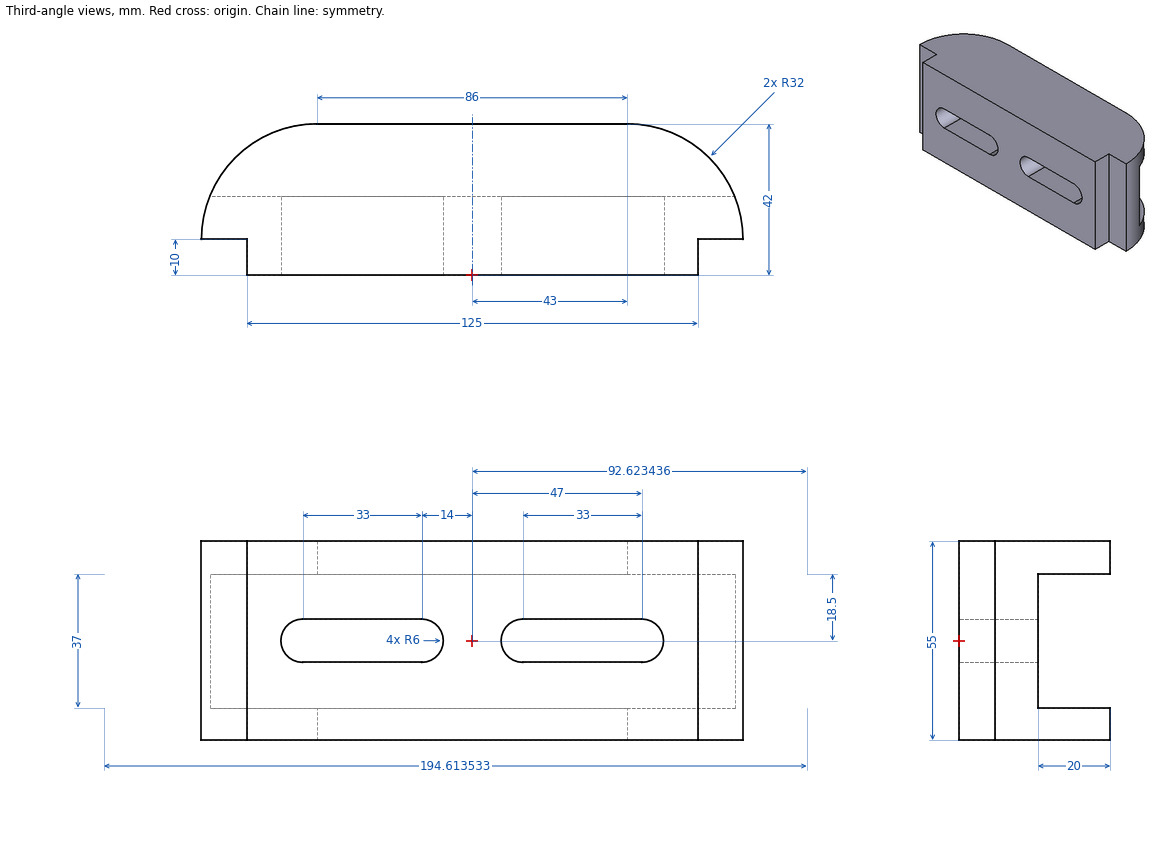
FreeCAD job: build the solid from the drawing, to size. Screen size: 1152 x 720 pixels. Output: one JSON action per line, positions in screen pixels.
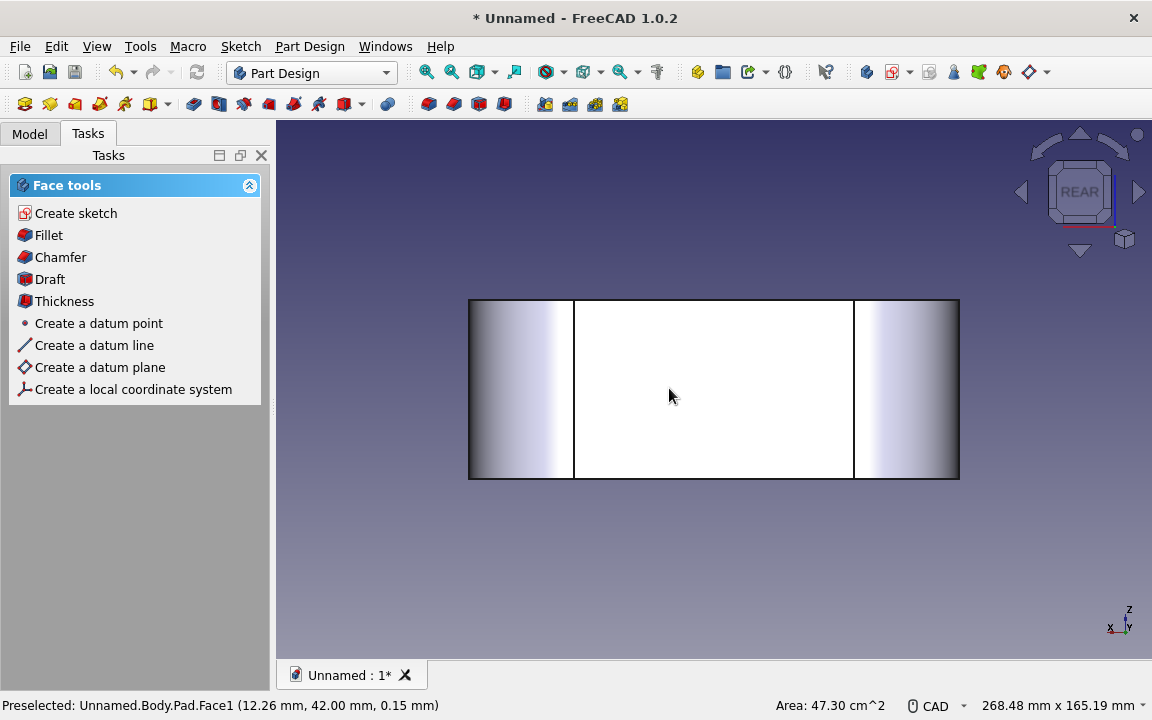
{"action": "left_click", "coordinate": [892, 72]}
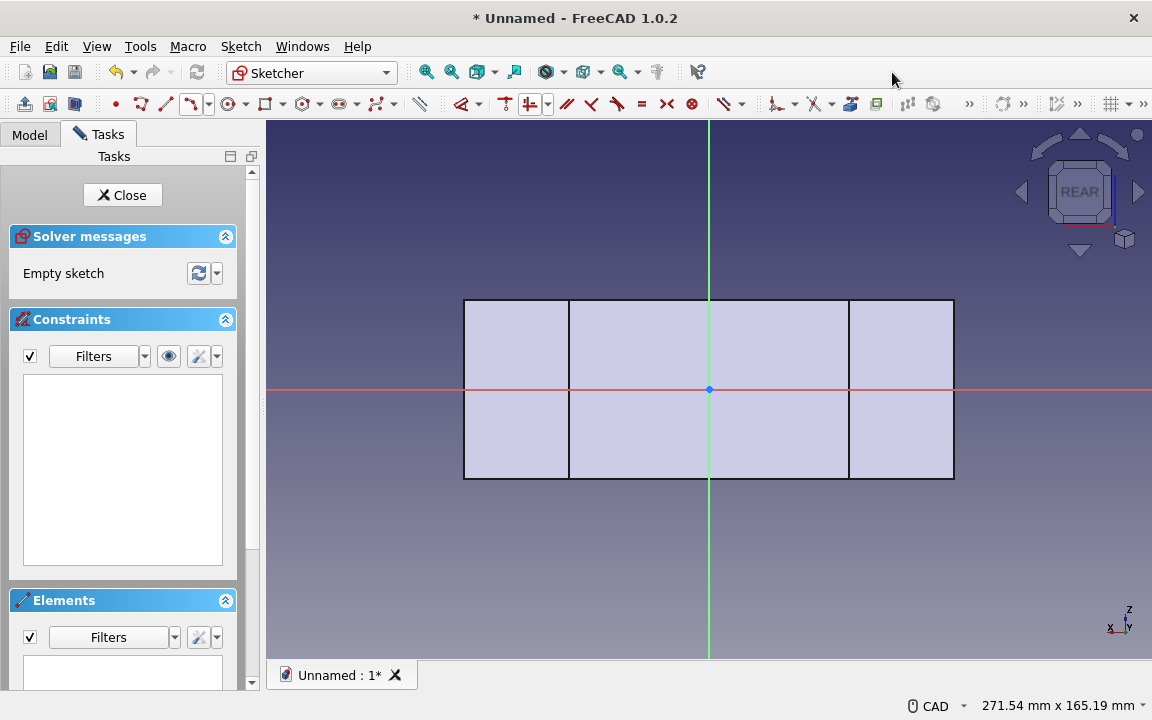
{"action": "scroll", "coordinate": [294, 390], "scroll_direction": "down", "scroll_amount": 1}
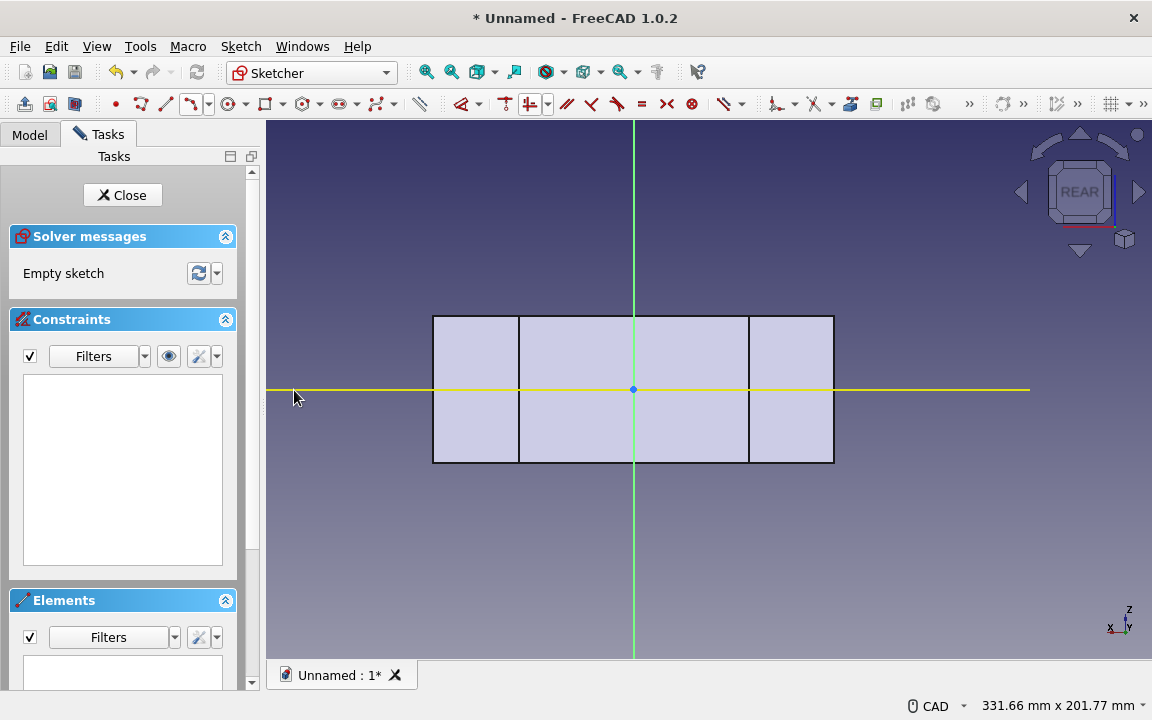
{"action": "left_click", "coordinate": [264, 104]}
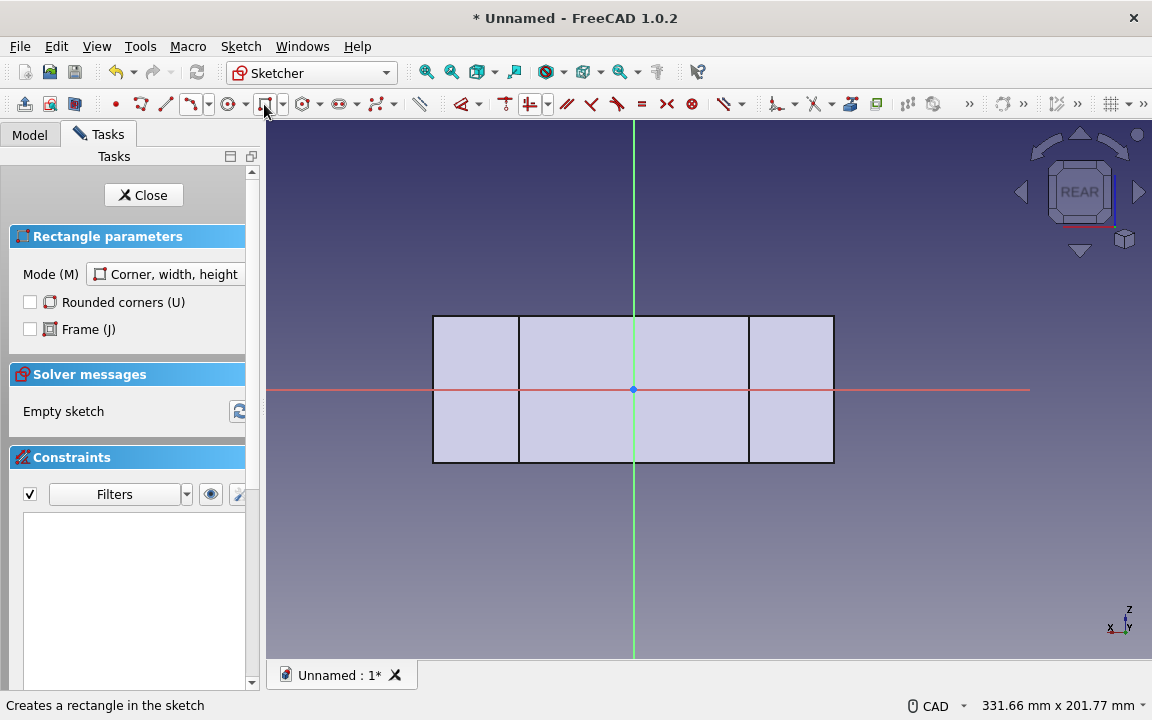
{"action": "left_click", "coordinate": [386, 340]}
{"action": "mouse_move", "coordinate": [906, 439]}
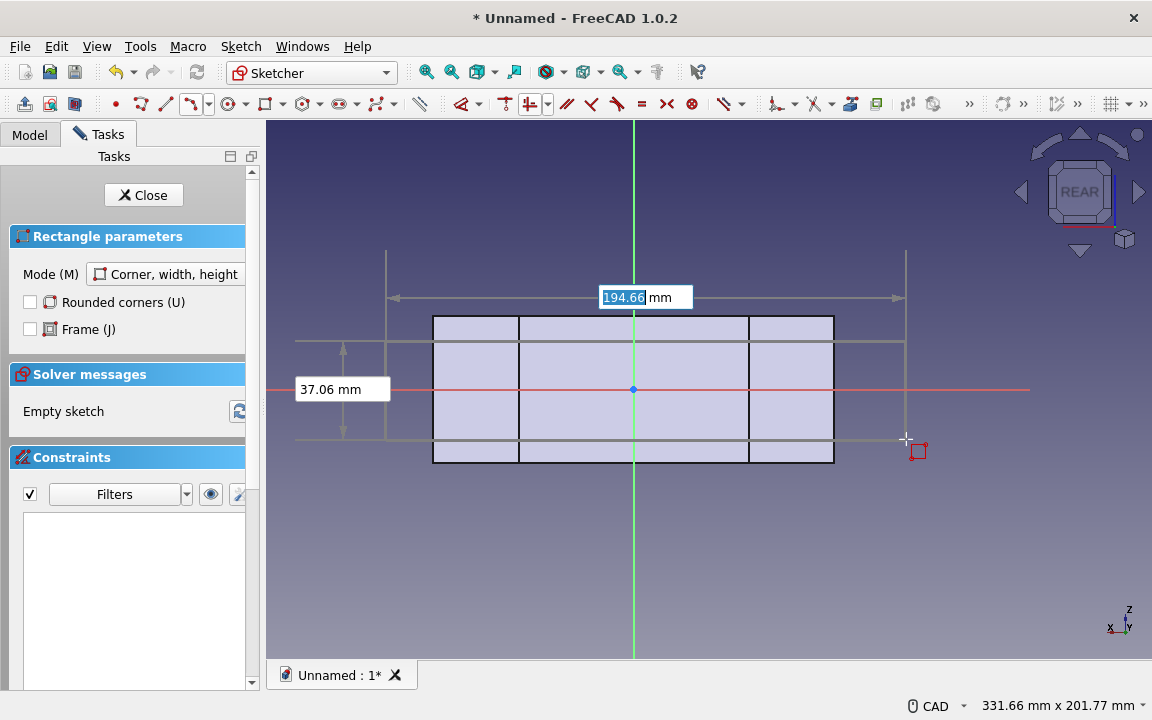
{"action": "type", "text": "194.613533"}
{"action": "key", "text": "Tab"}
{"action": "type", "text": "37"}
{"action": "key", "text": "Return"}
{"action": "key", "text": "Escape"}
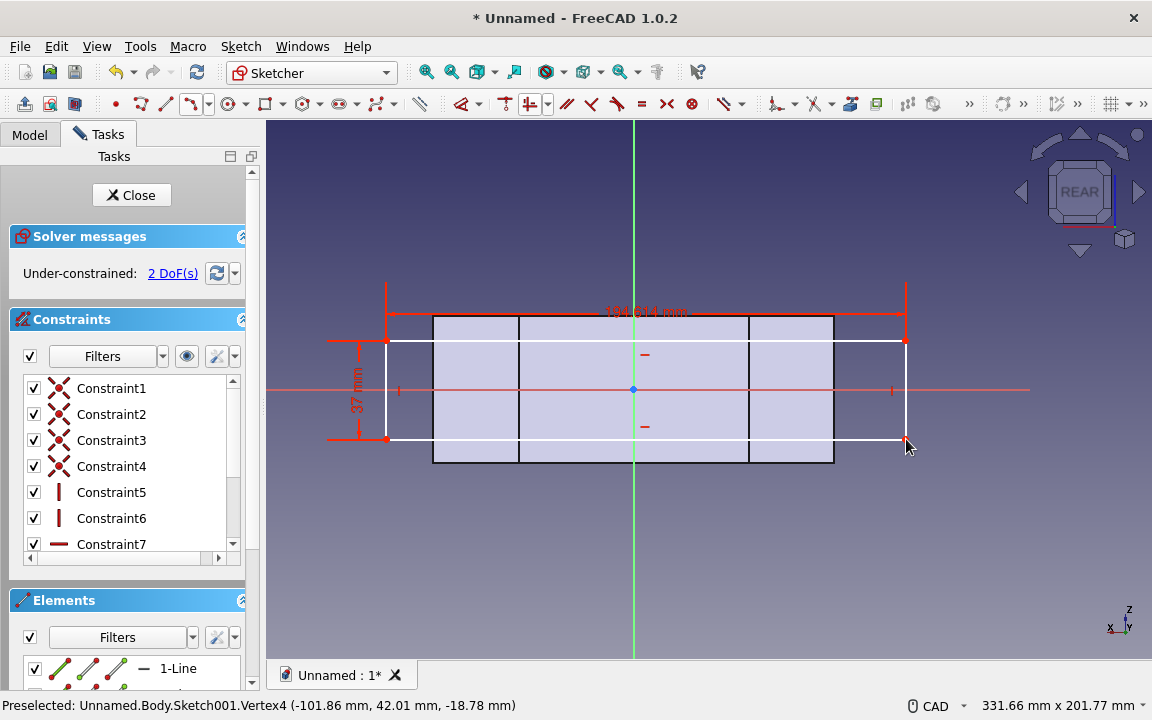
{"action": "left_click", "coordinate": [460, 104]}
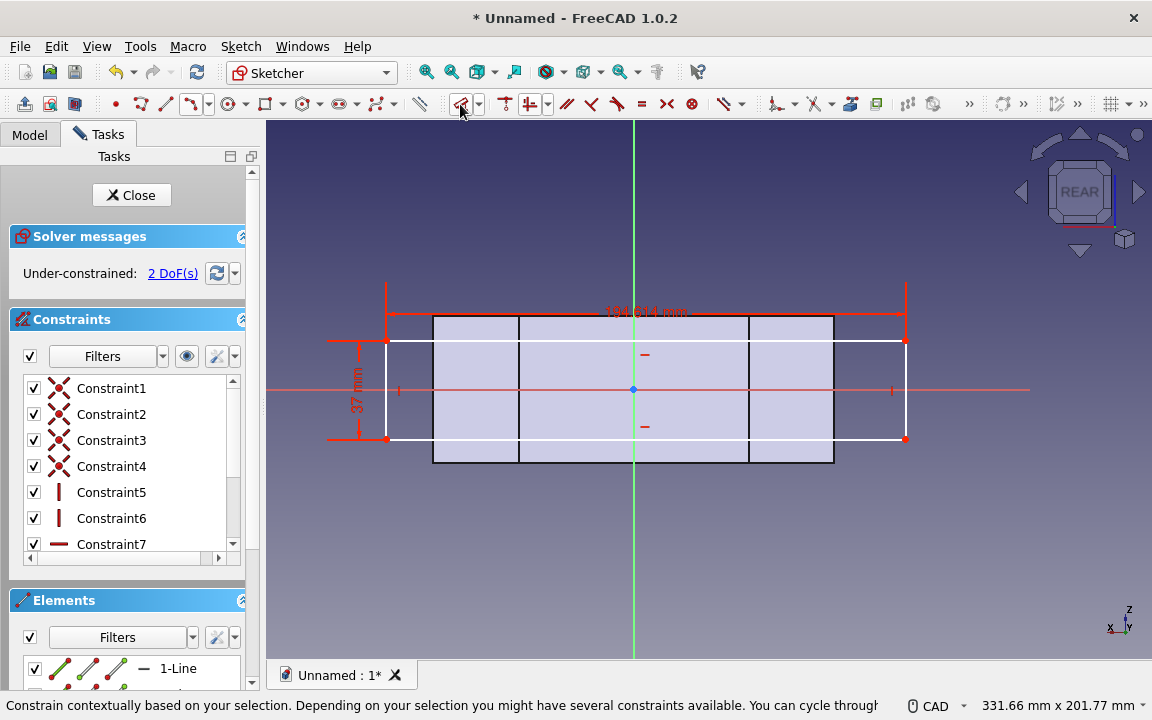
{"action": "left_click", "coordinate": [386, 341]}
{"action": "left_click", "coordinate": [352, 365]}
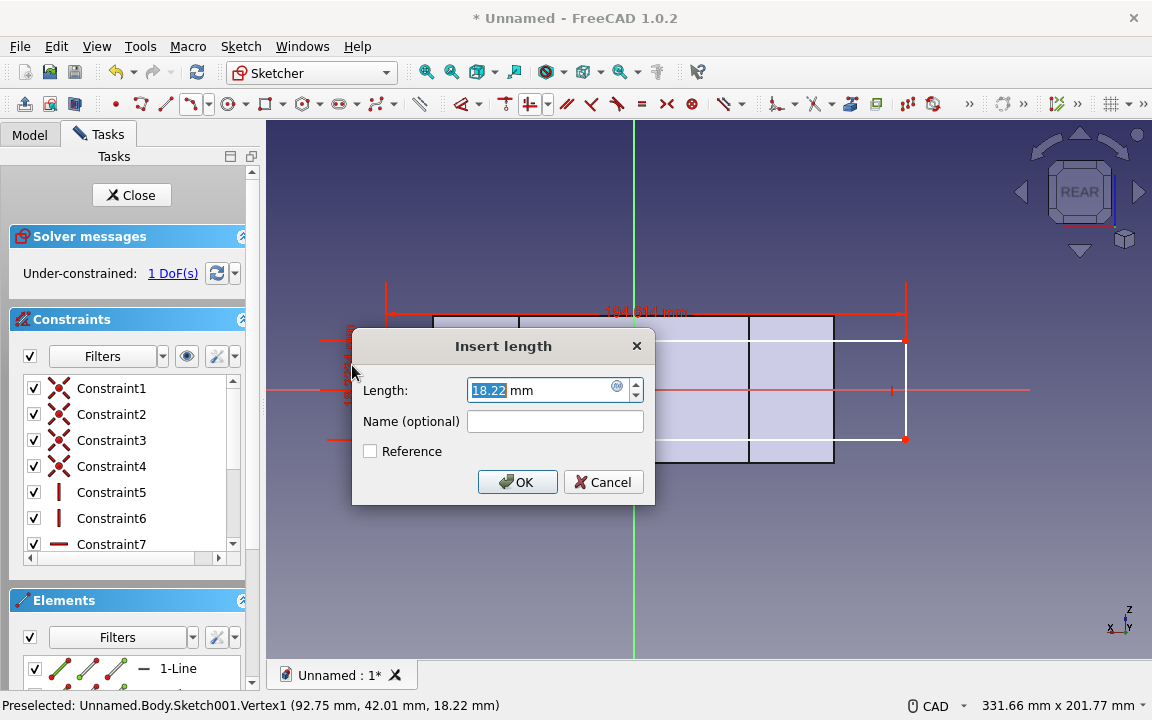
{"action": "type", "text": "18.5"}
{"action": "key", "text": "Return"}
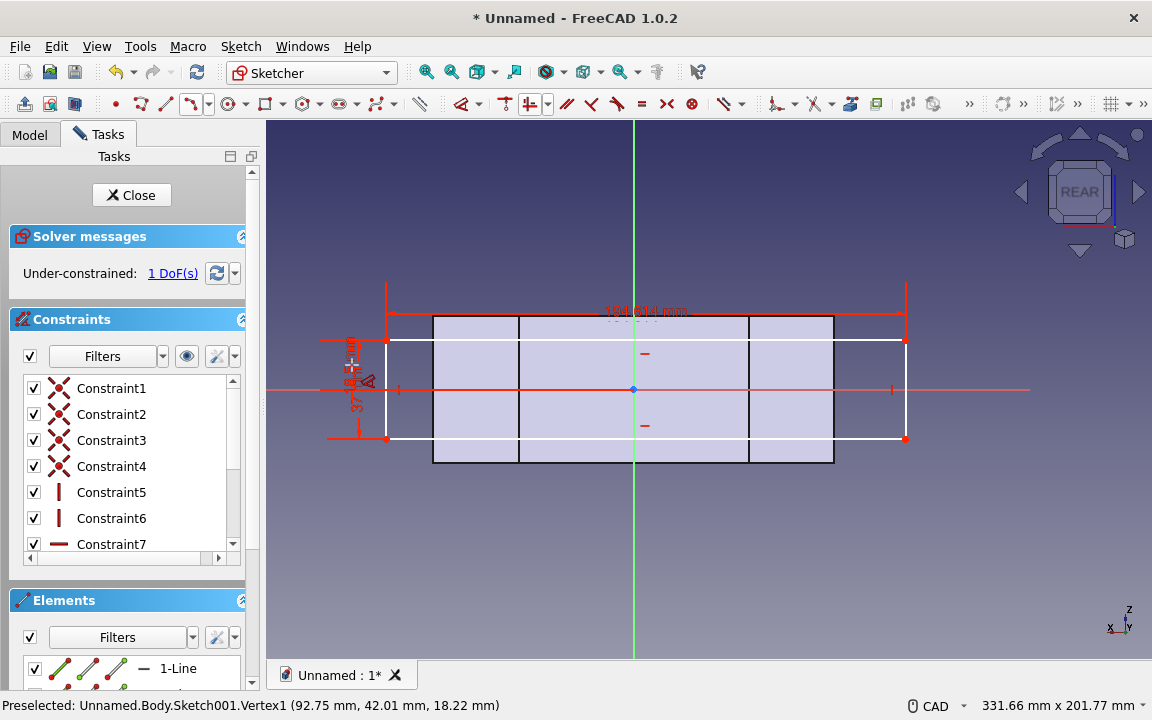
{"action": "left_click", "coordinate": [386, 340]}
{"action": "left_click", "coordinate": [510, 306]}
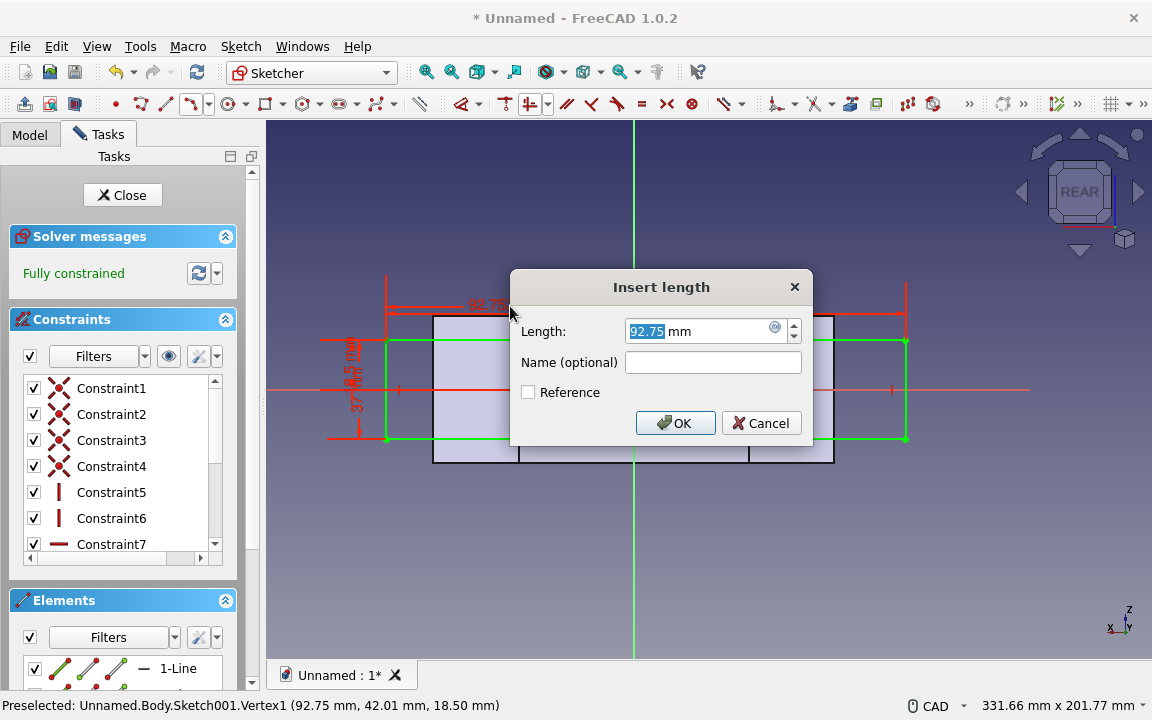
{"action": "type", "text": "92.623436"}
{"action": "key", "text": "Return"}
{"action": "key", "text": "Escape"}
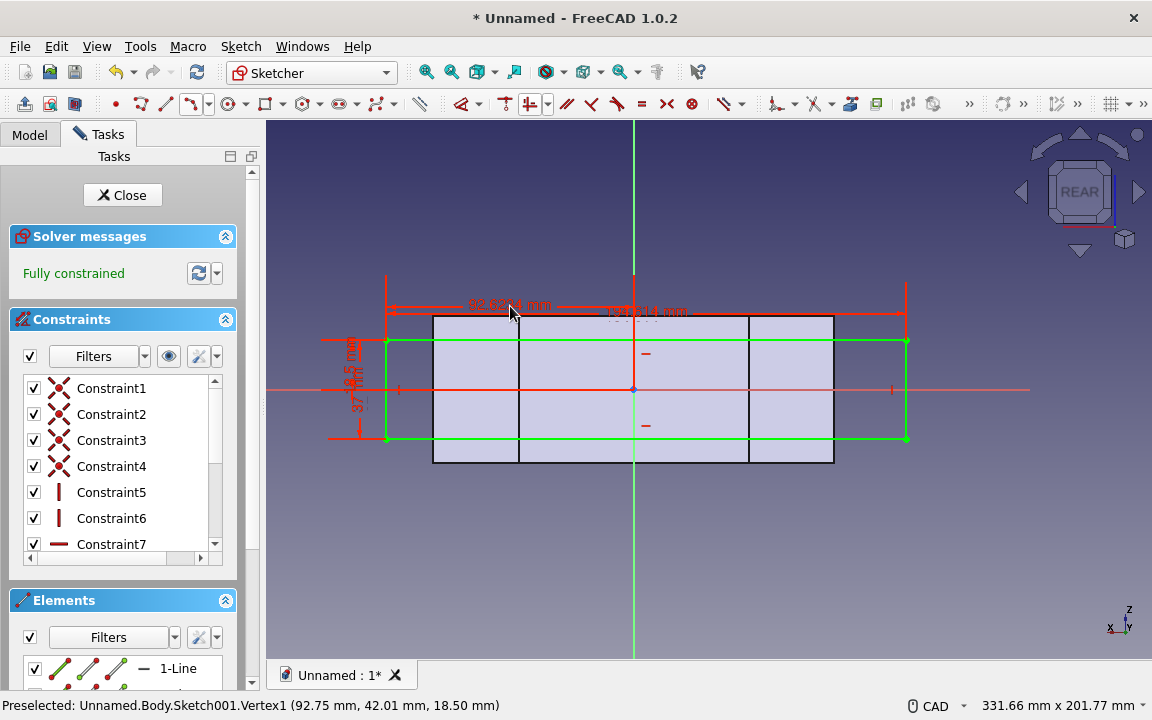
{"action": "left_click", "coordinate": [123, 195]}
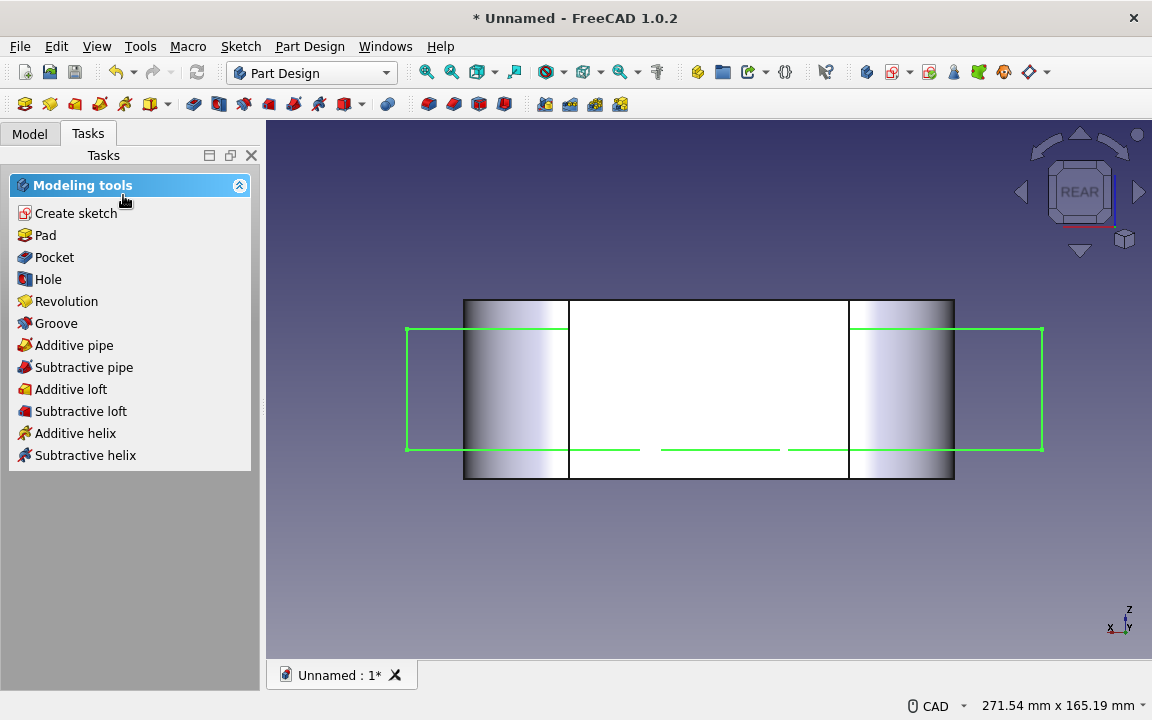
{"action": "left_click", "coordinate": [194, 104]}